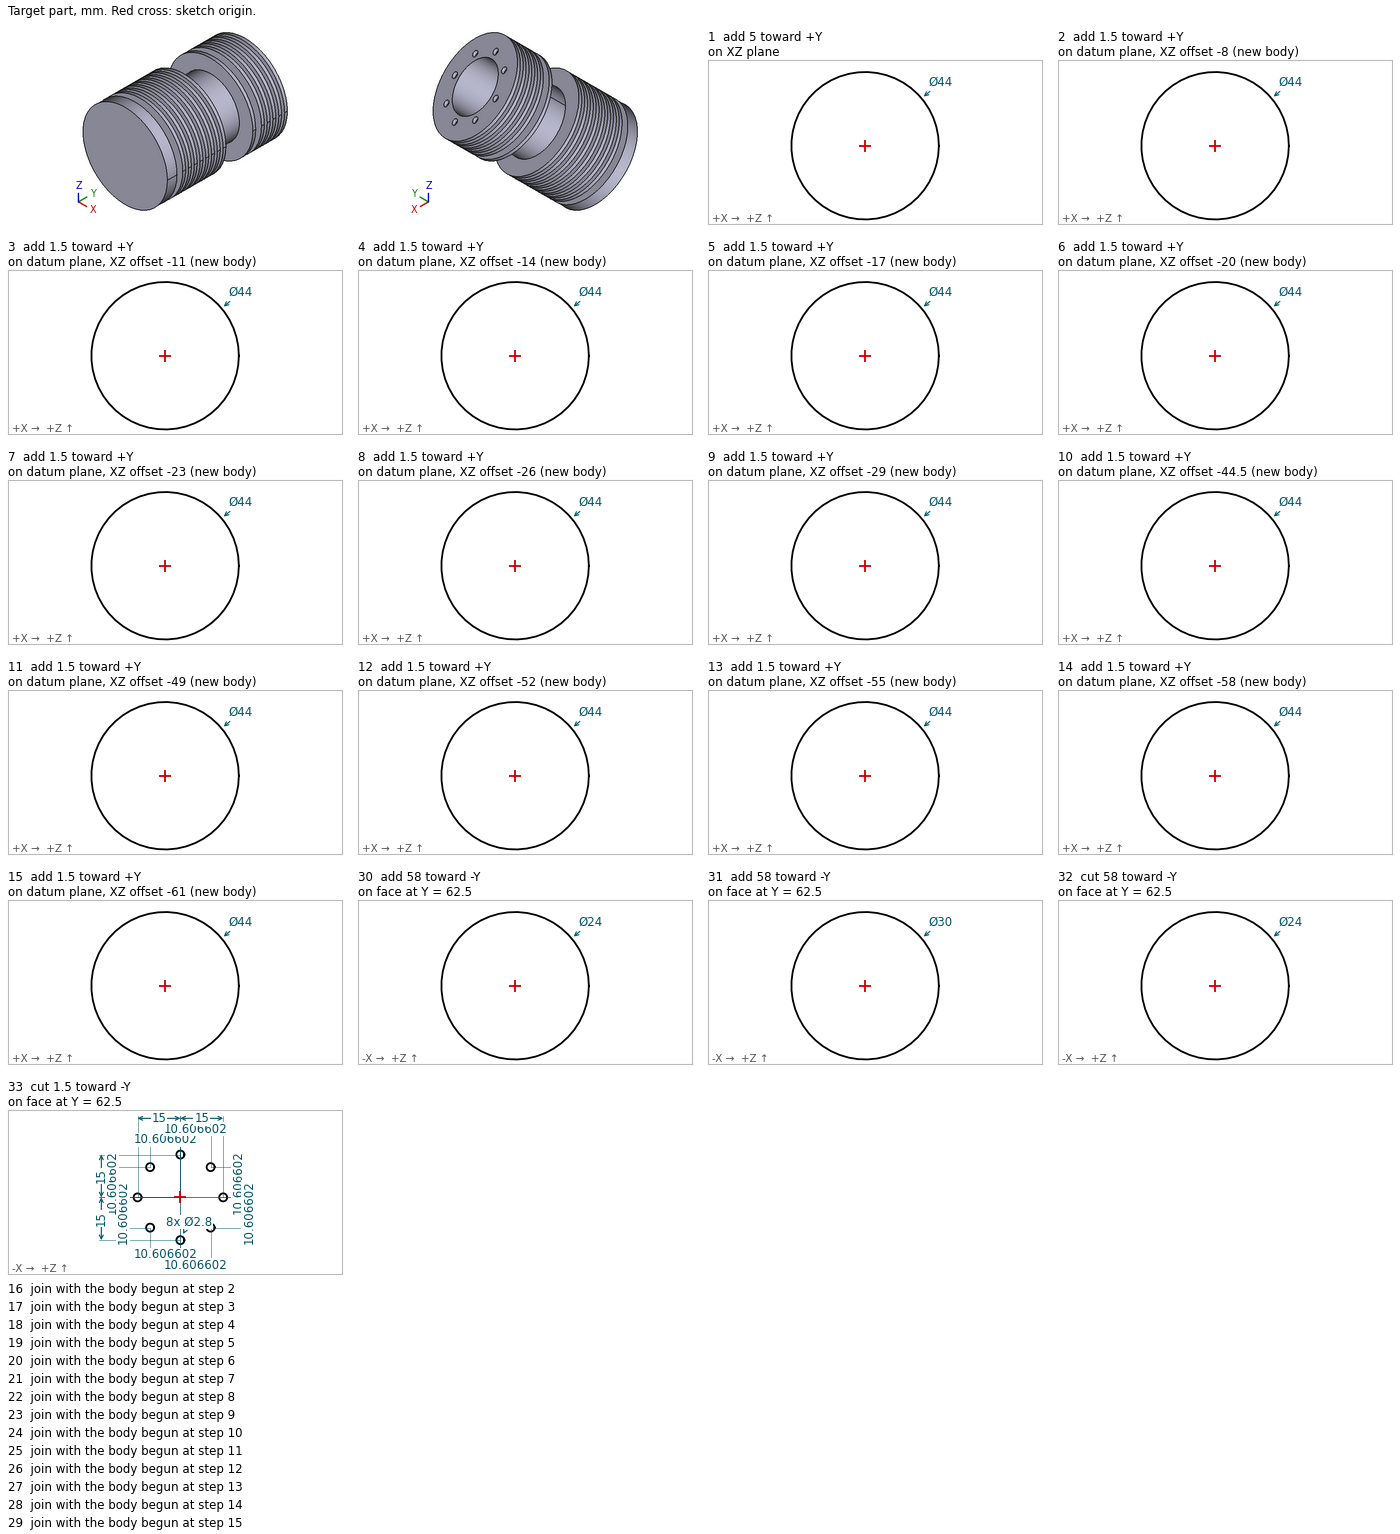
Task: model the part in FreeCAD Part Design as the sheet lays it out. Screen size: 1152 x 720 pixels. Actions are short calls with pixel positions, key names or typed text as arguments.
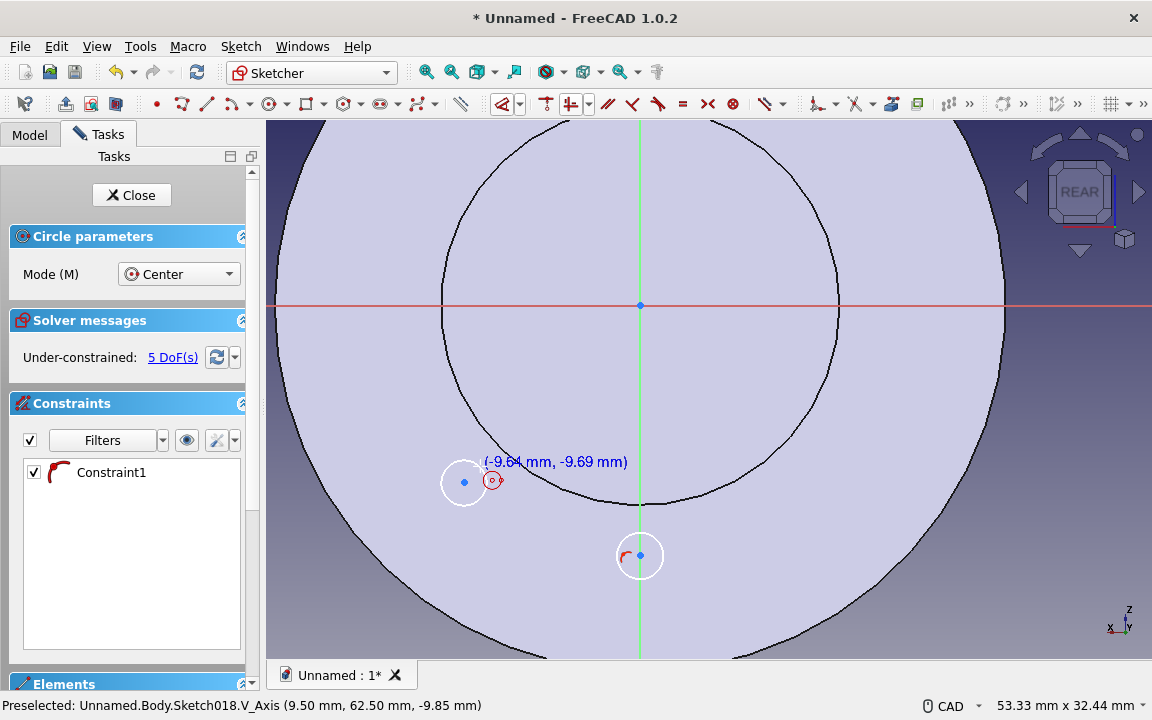
click(391, 306)
click(407, 290)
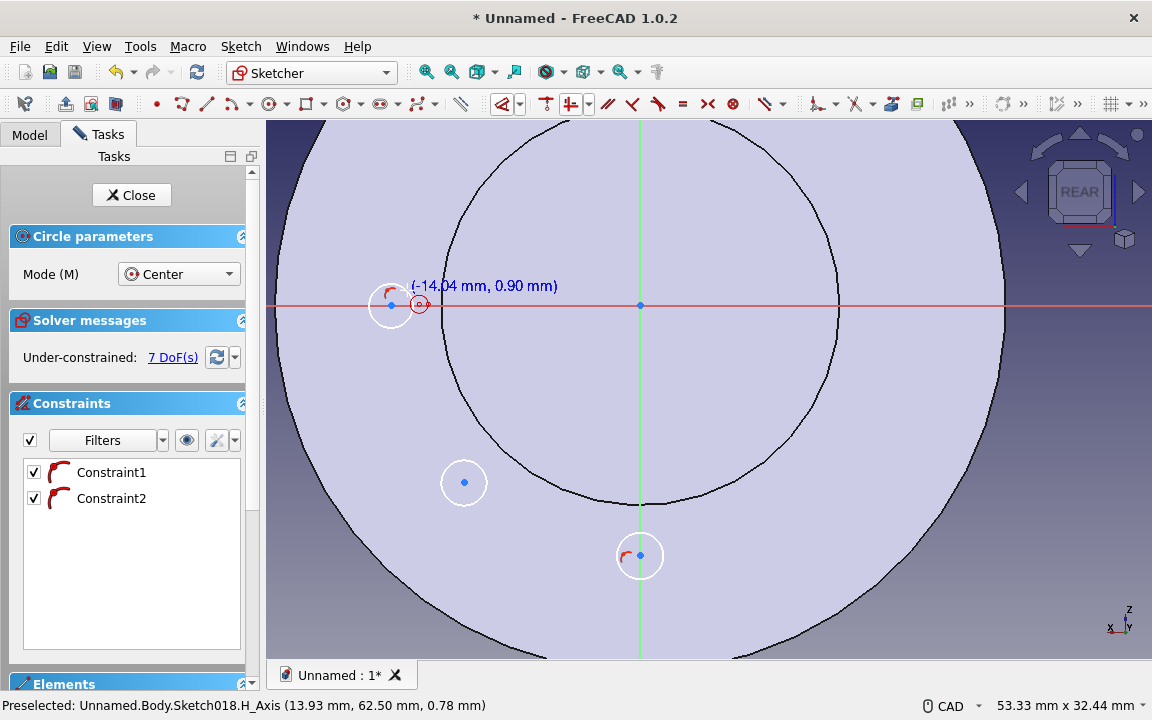
scroll(641, 559, down, 2)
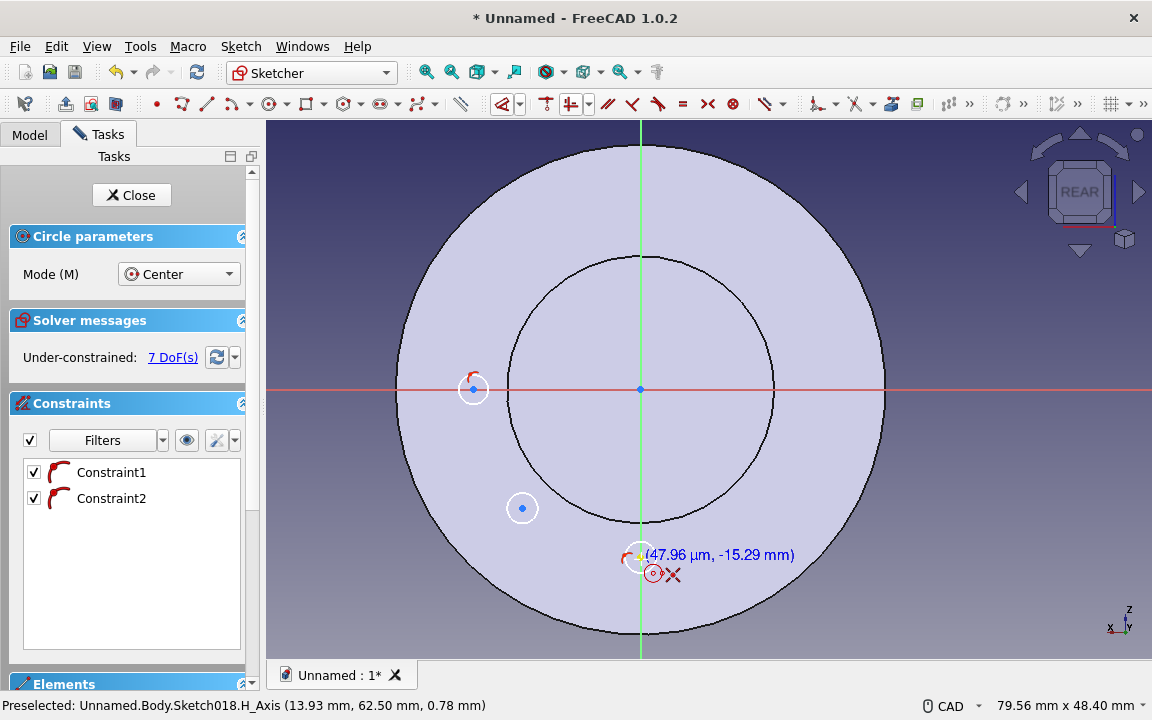
scroll(522, 272, up, 2)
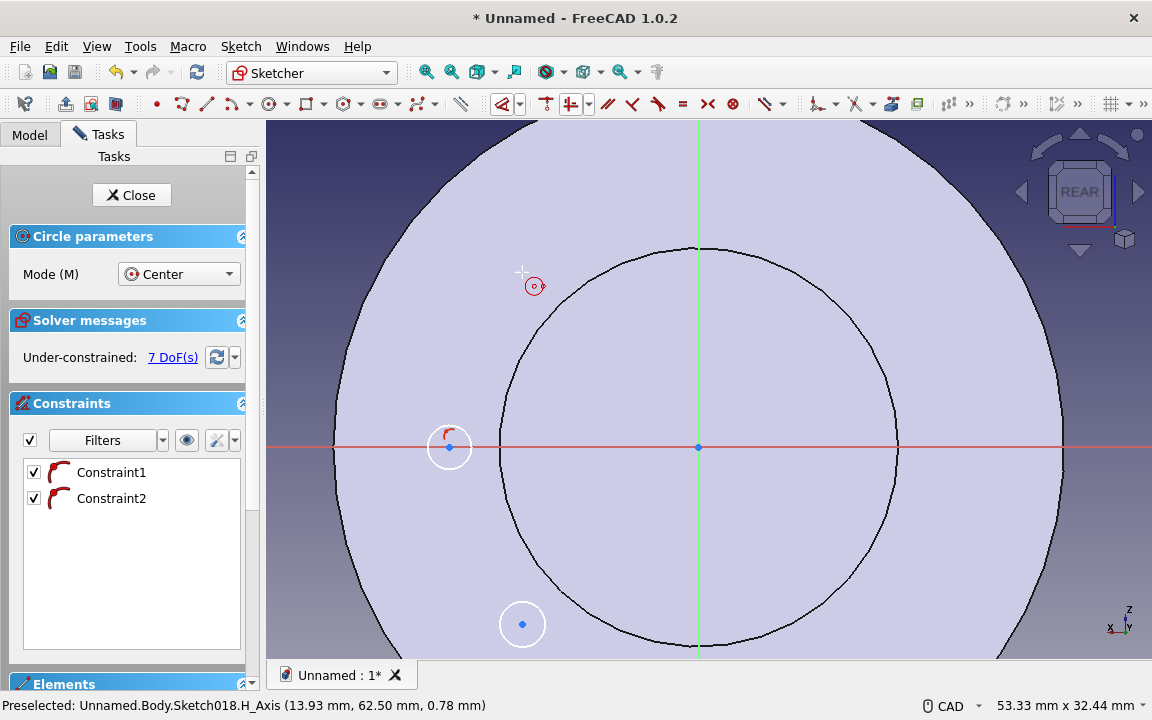
click(523, 271)
click(539, 255)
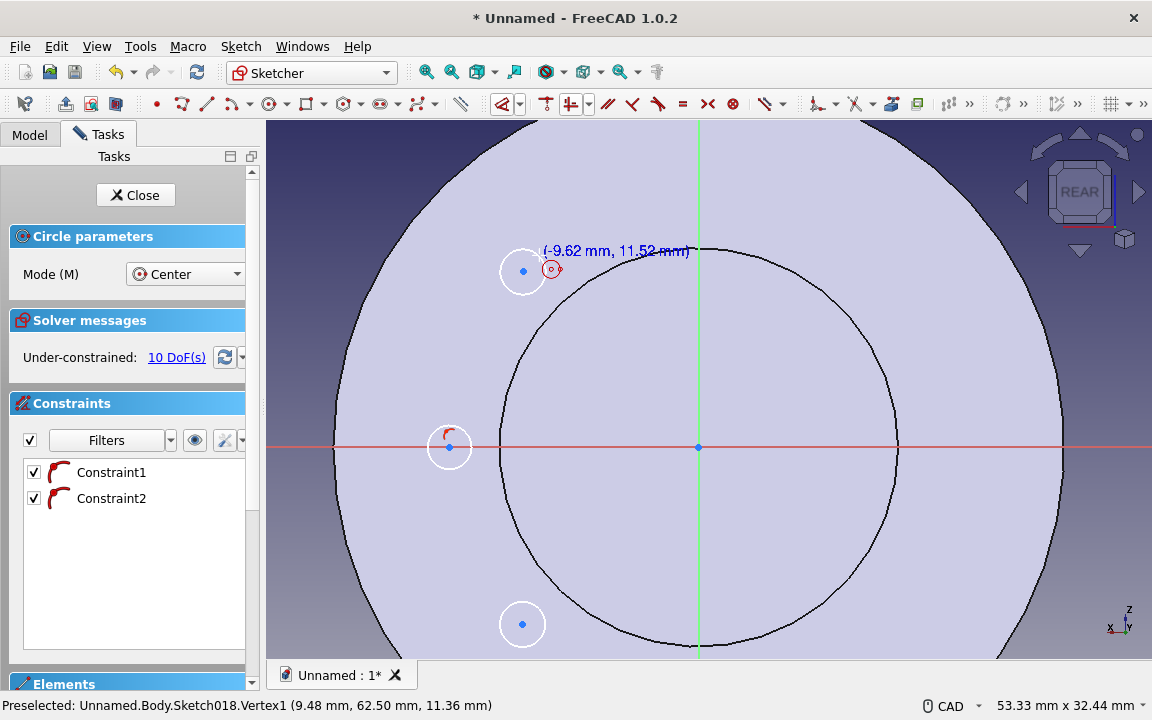
click(699, 198)
click(715, 182)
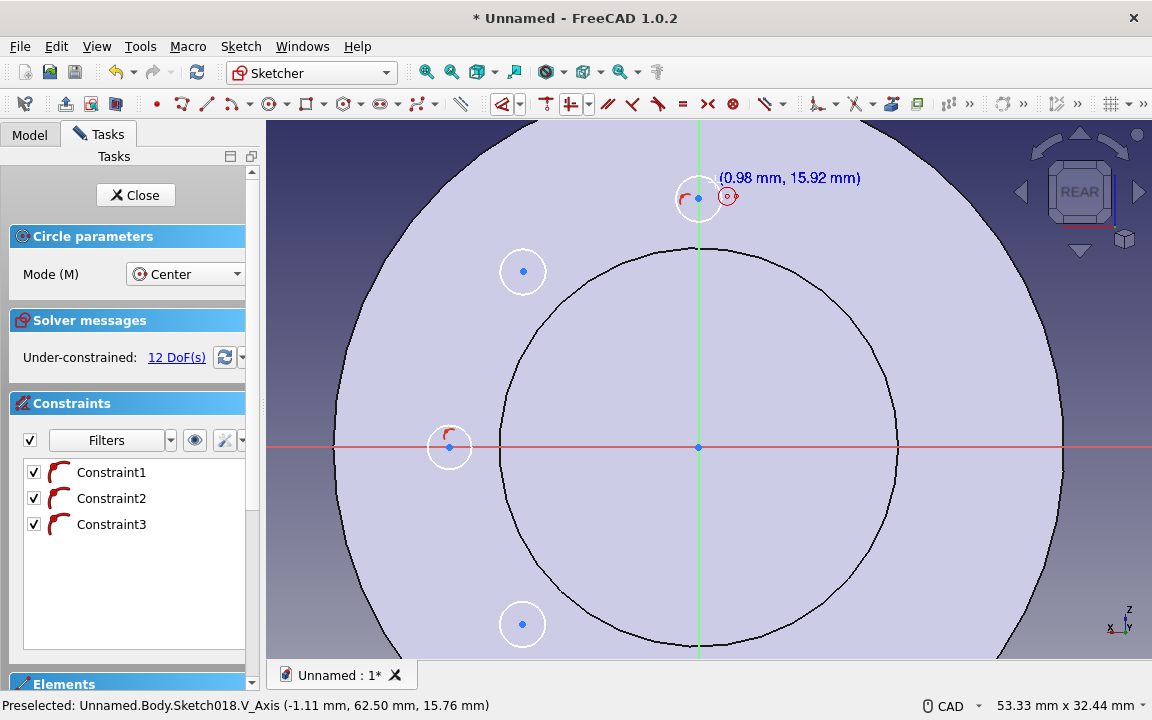
click(875, 271)
click(891, 255)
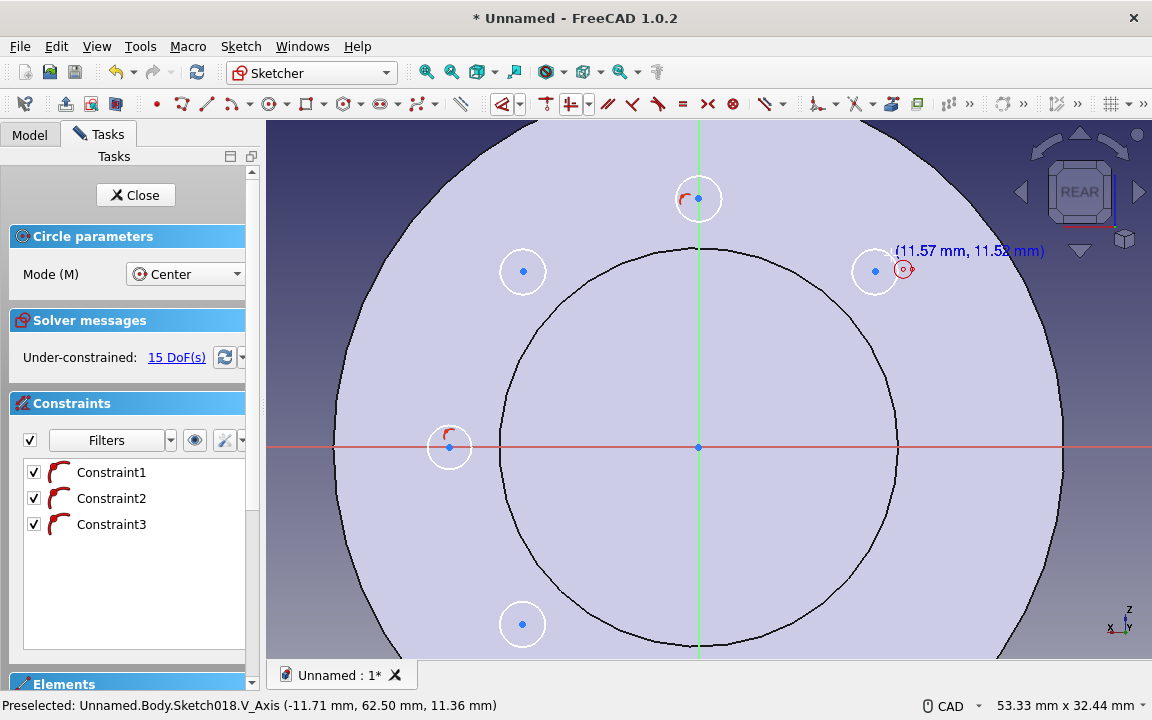
click(948, 447)
click(964, 431)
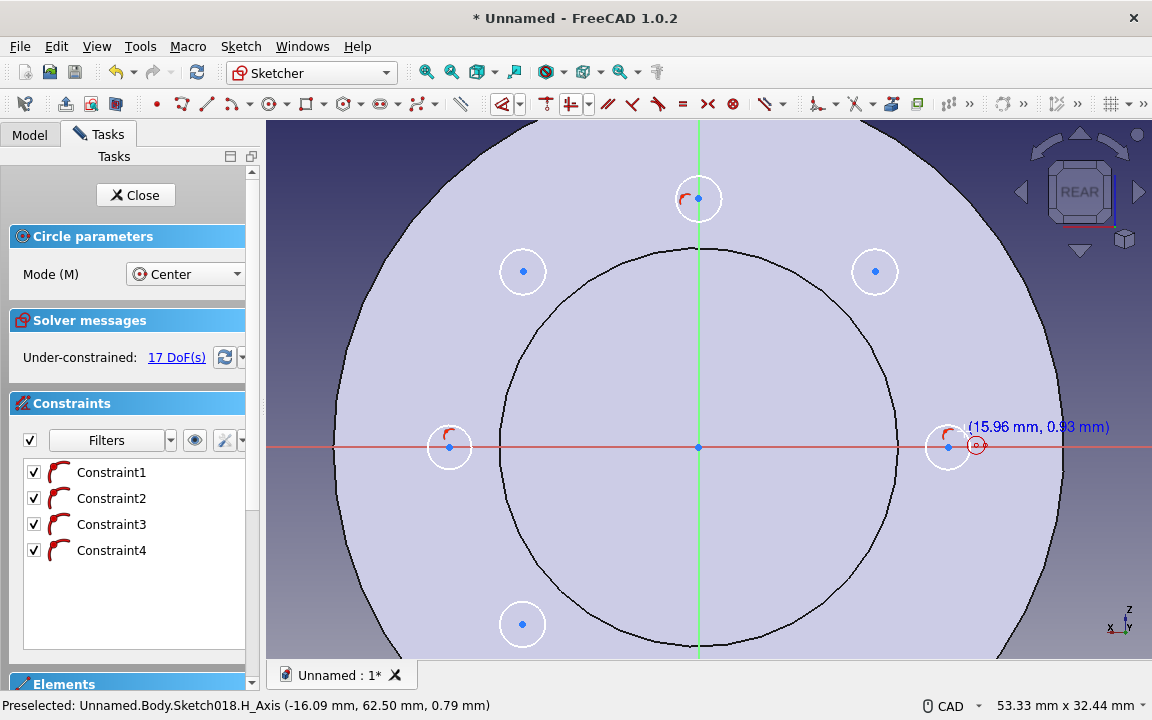
click(875, 624)
click(891, 607)
key(Escape)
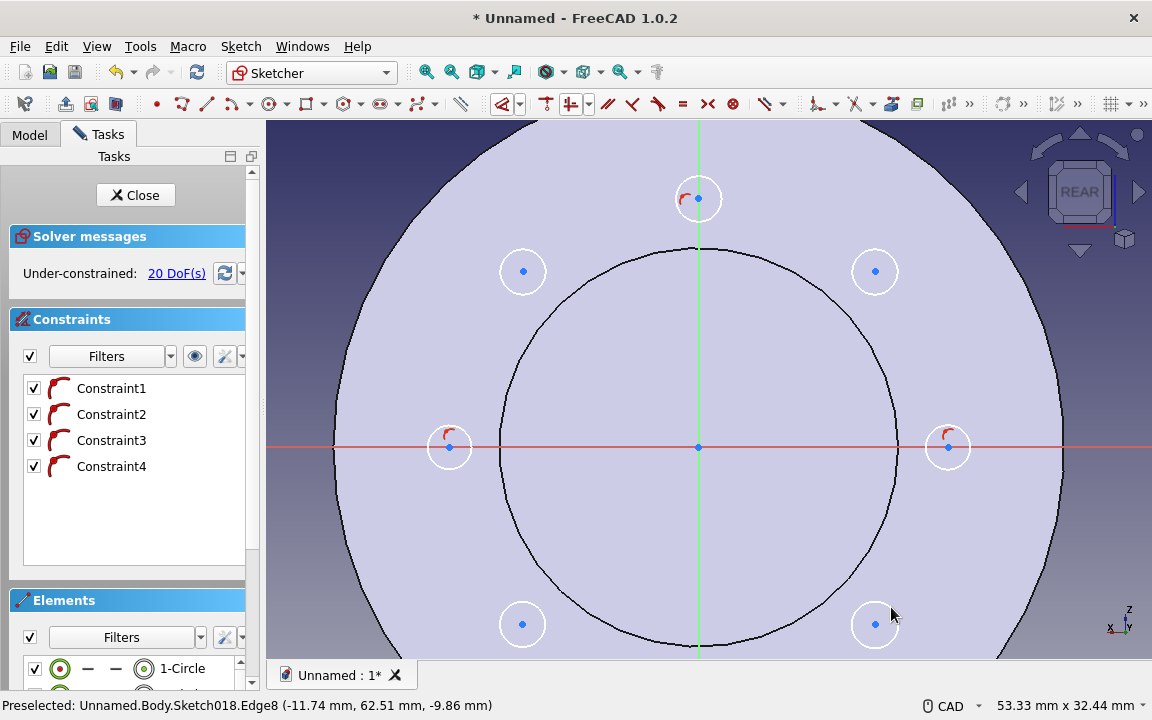
scroll(522, 272, down, 2)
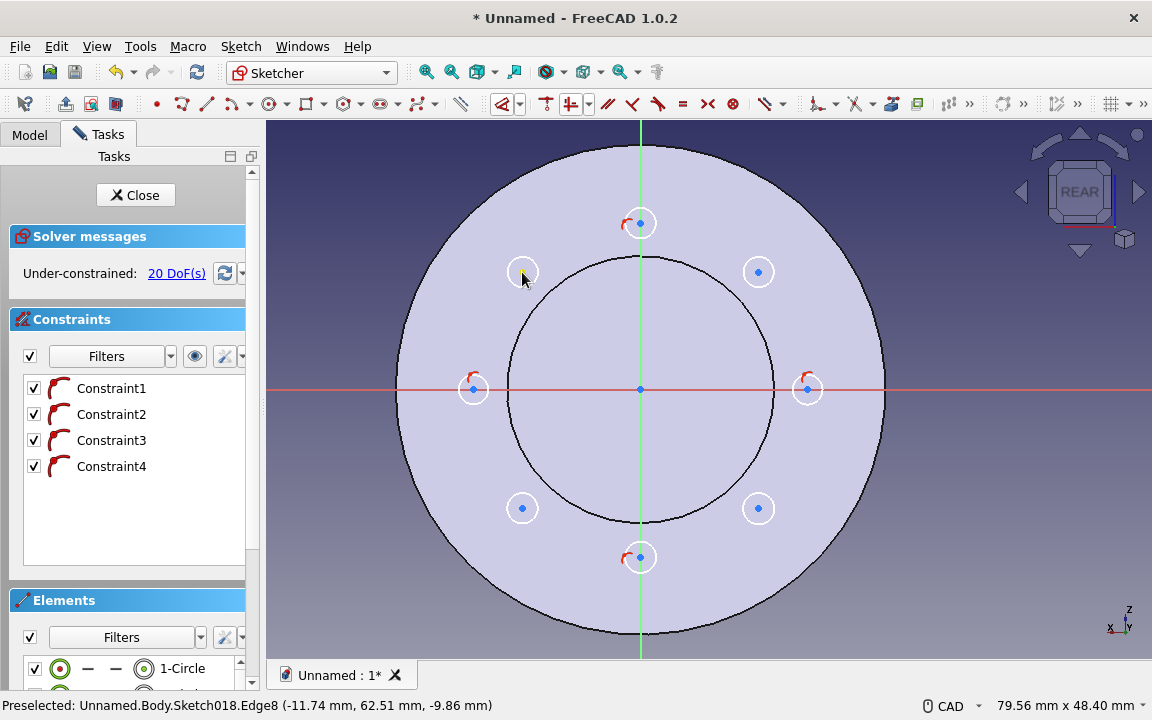
scroll(652, 546, up, 2)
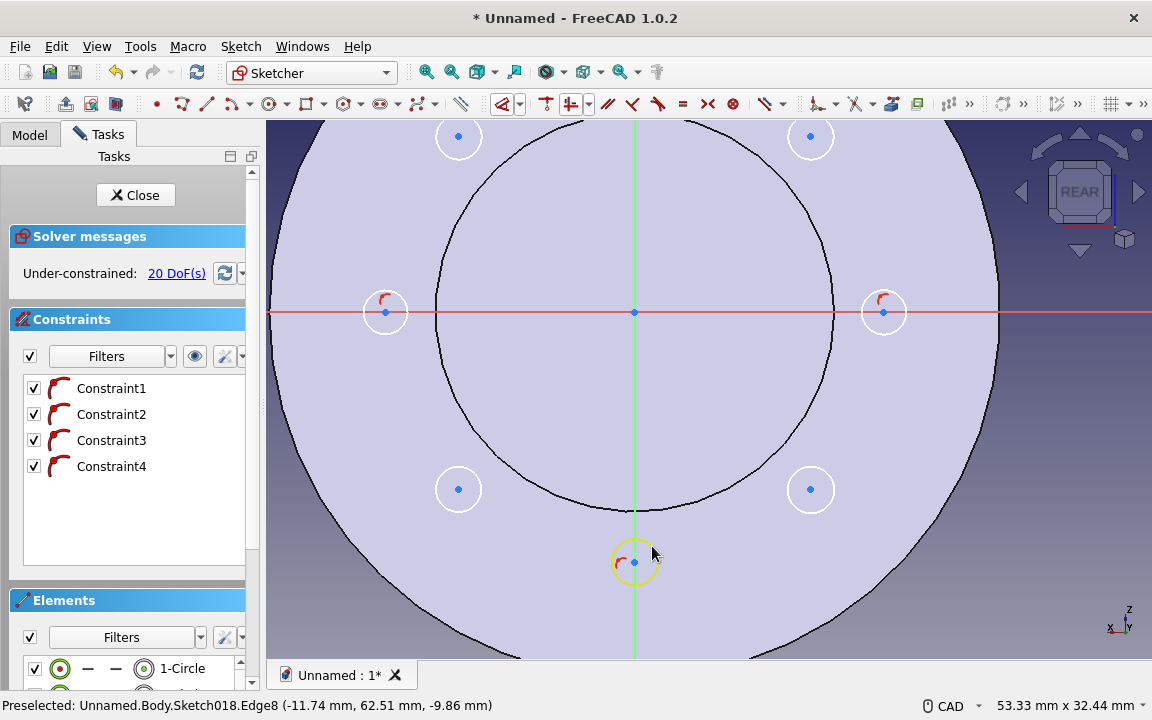
click(651, 546)